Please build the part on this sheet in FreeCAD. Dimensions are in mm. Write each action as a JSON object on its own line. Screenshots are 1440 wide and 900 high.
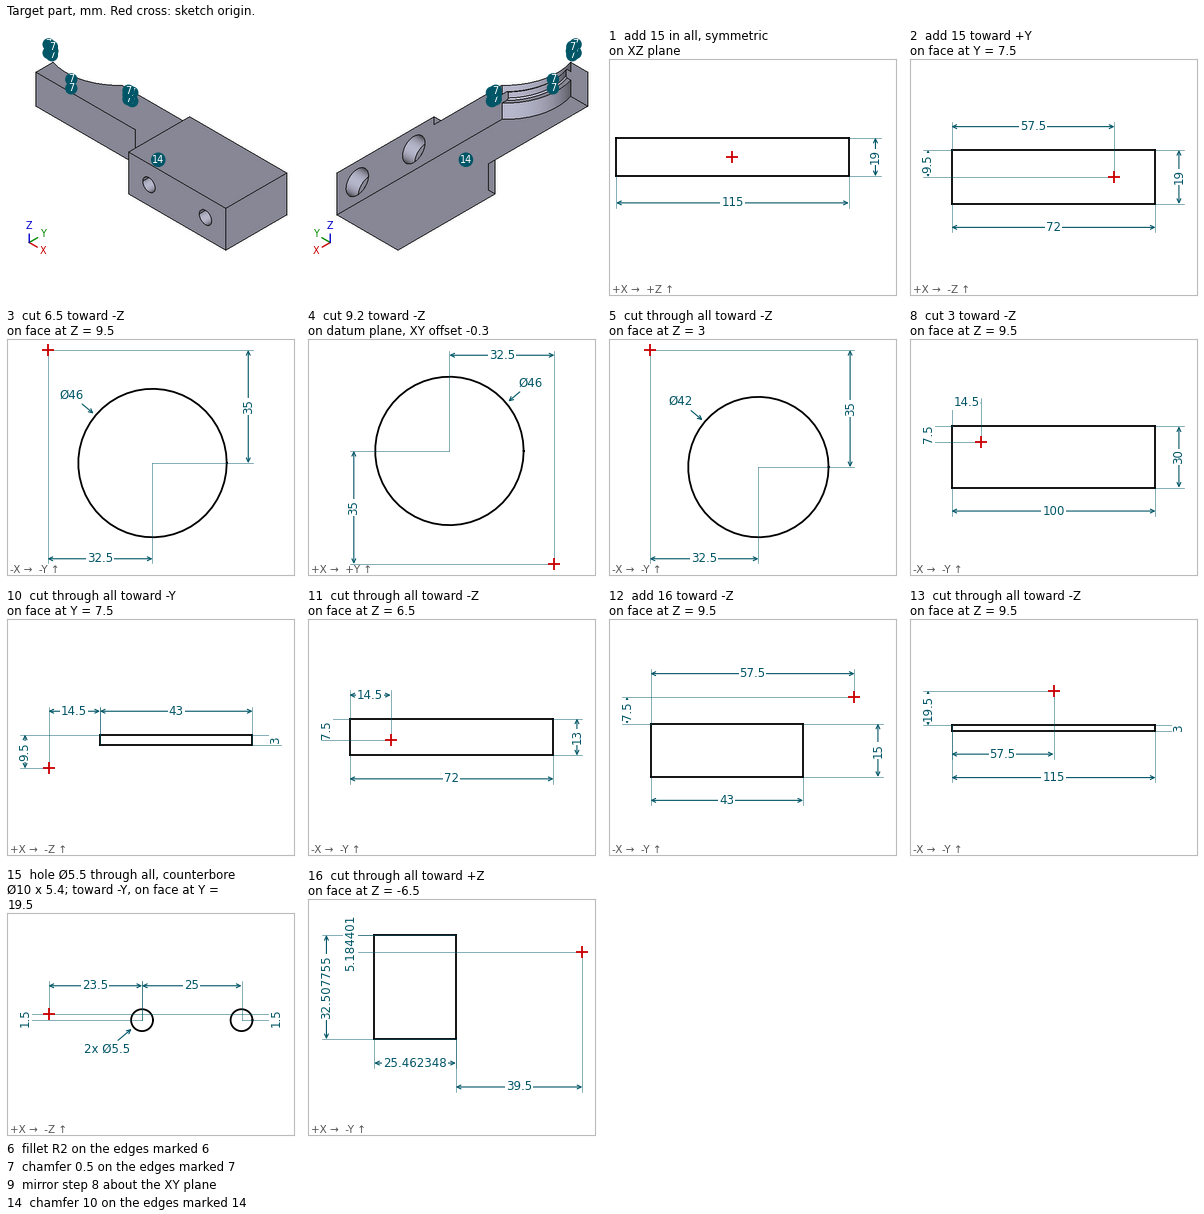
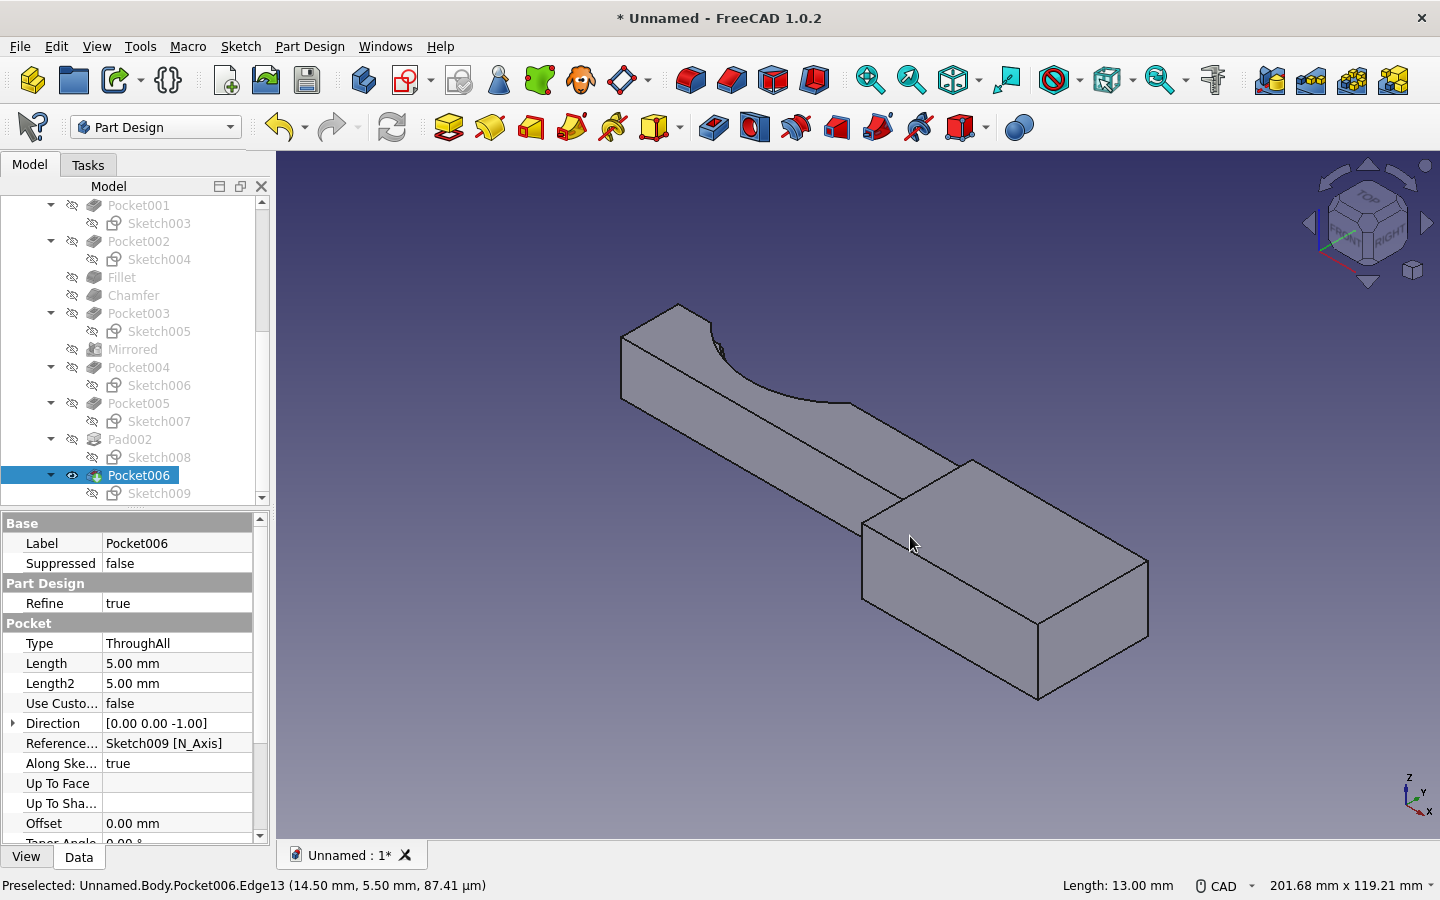
{"action": "left_click", "coordinate": [732, 80]}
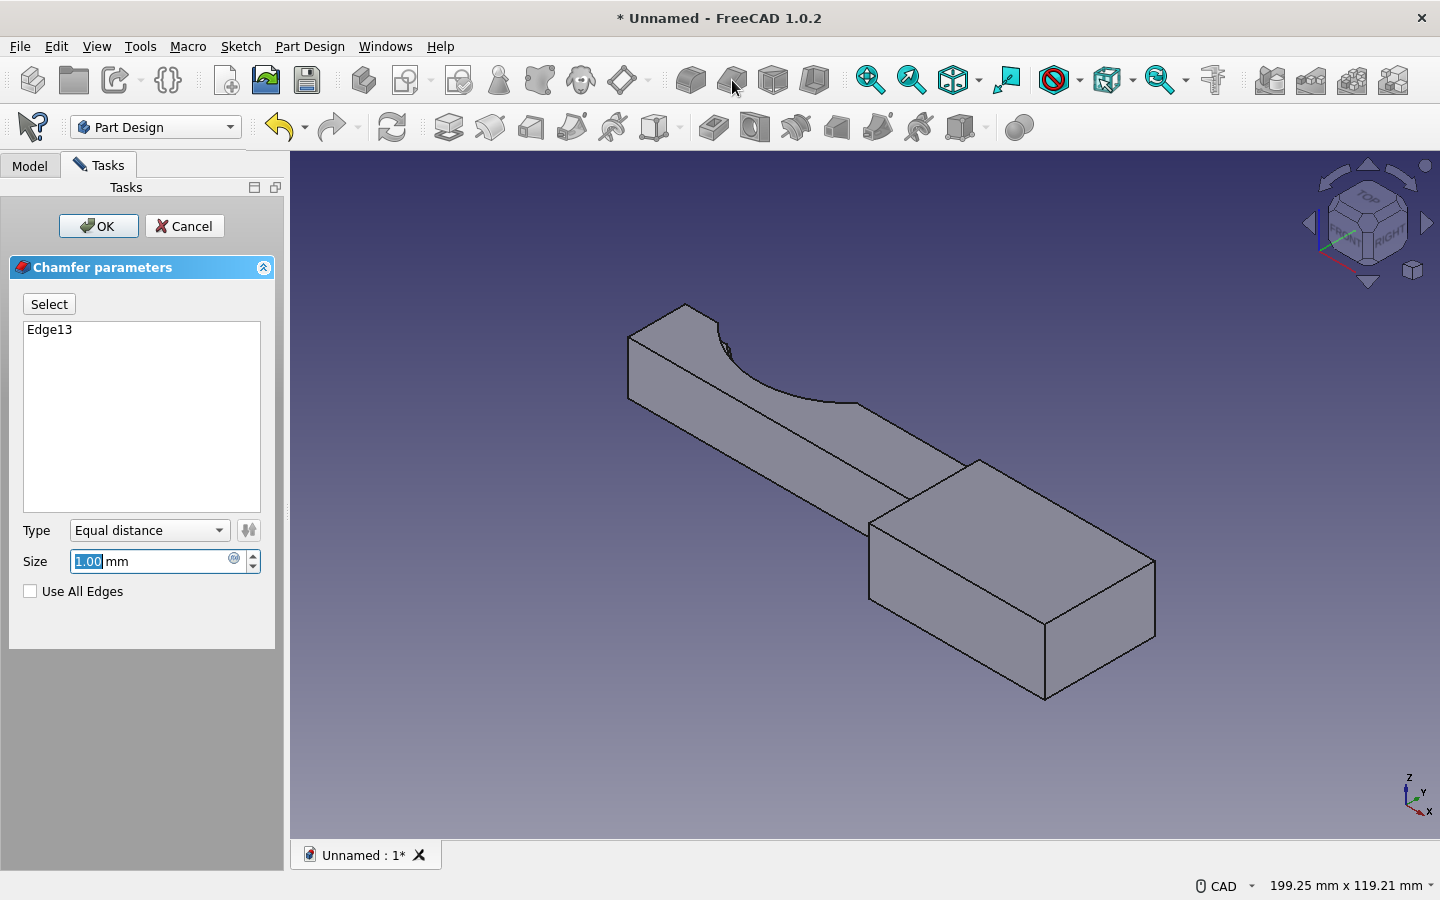
{"action": "type", "text": "10"}
{"action": "key", "text": "Tab"}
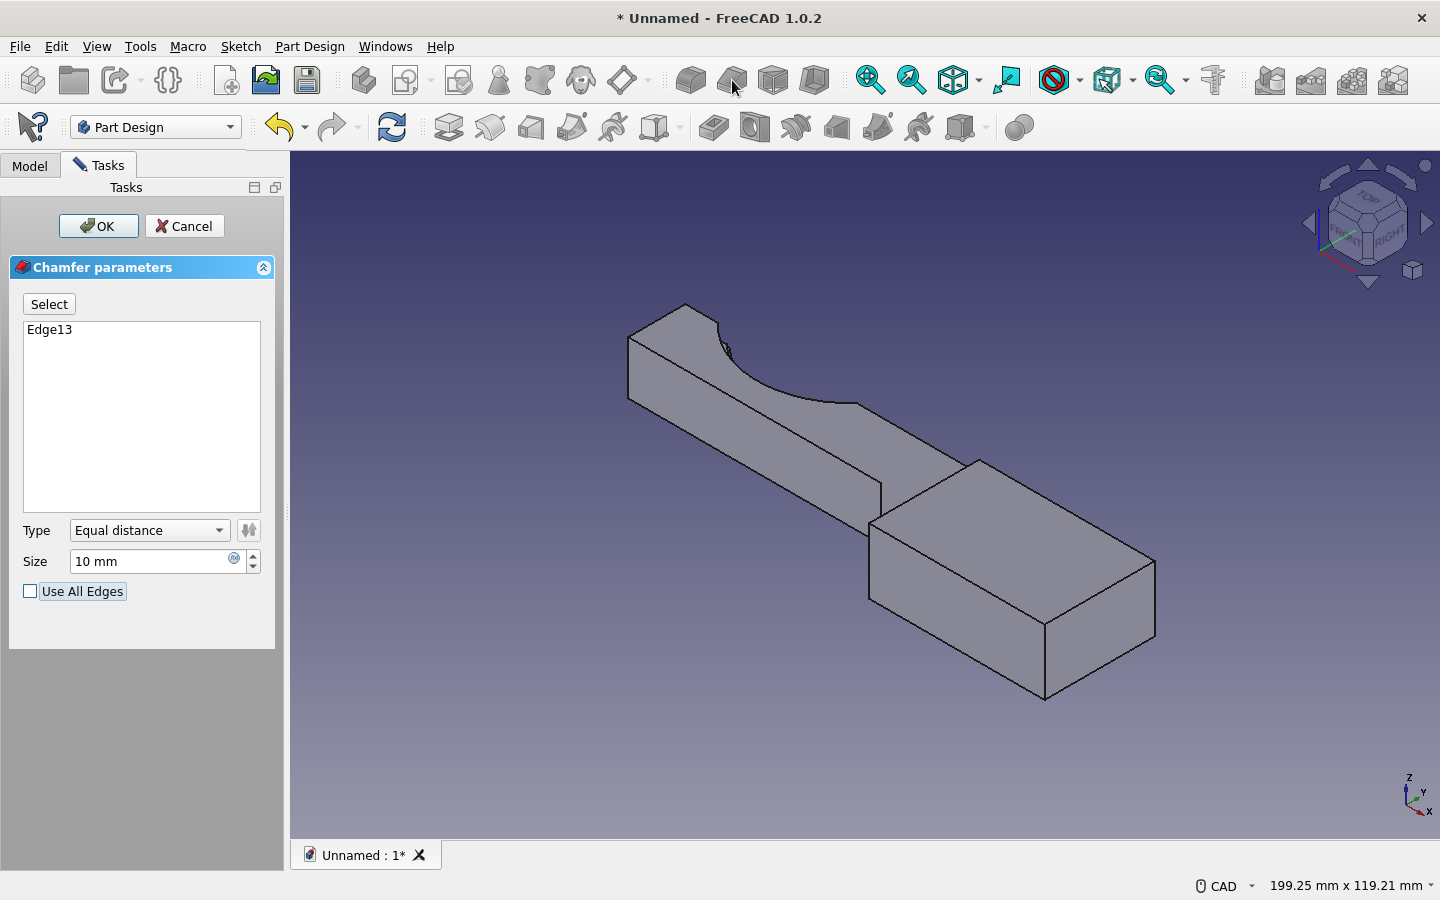
{"action": "left_click", "coordinate": [99, 226]}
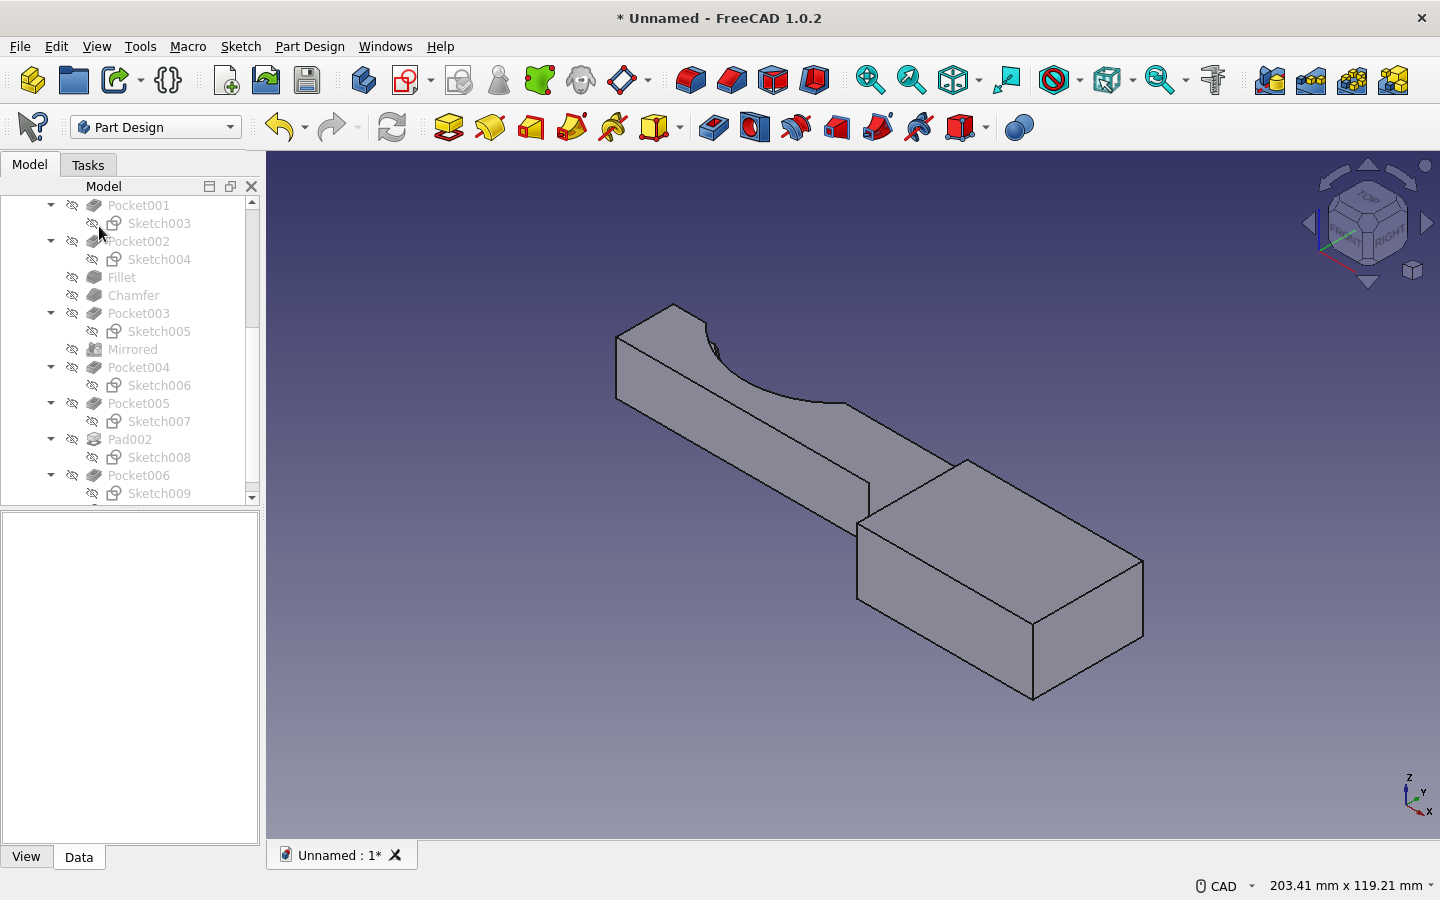
{"action": "key", "text": "4"}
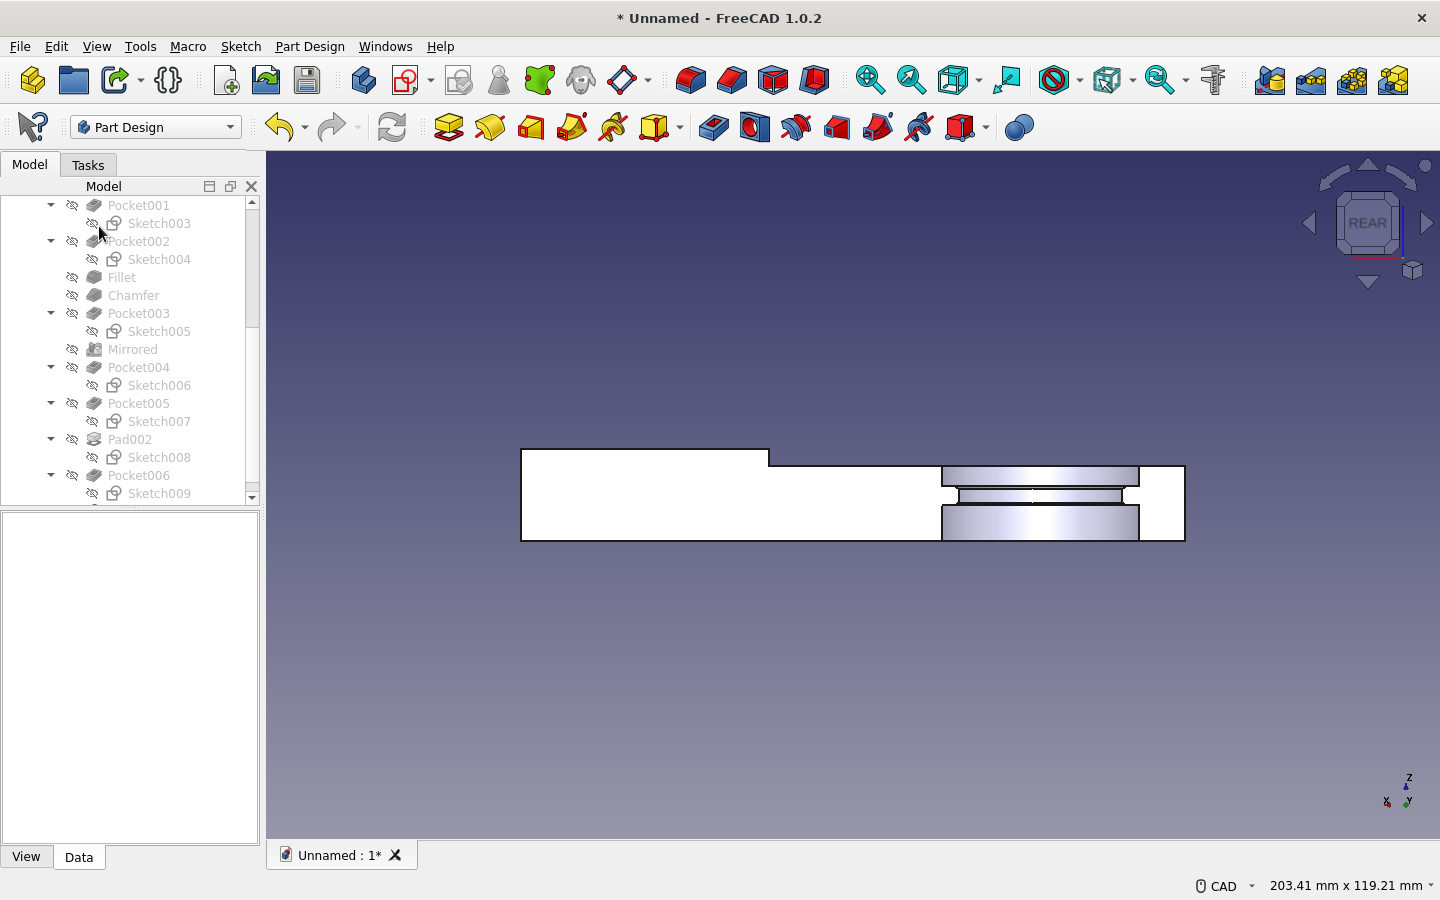
{"action": "left_click", "coordinate": [615, 494]}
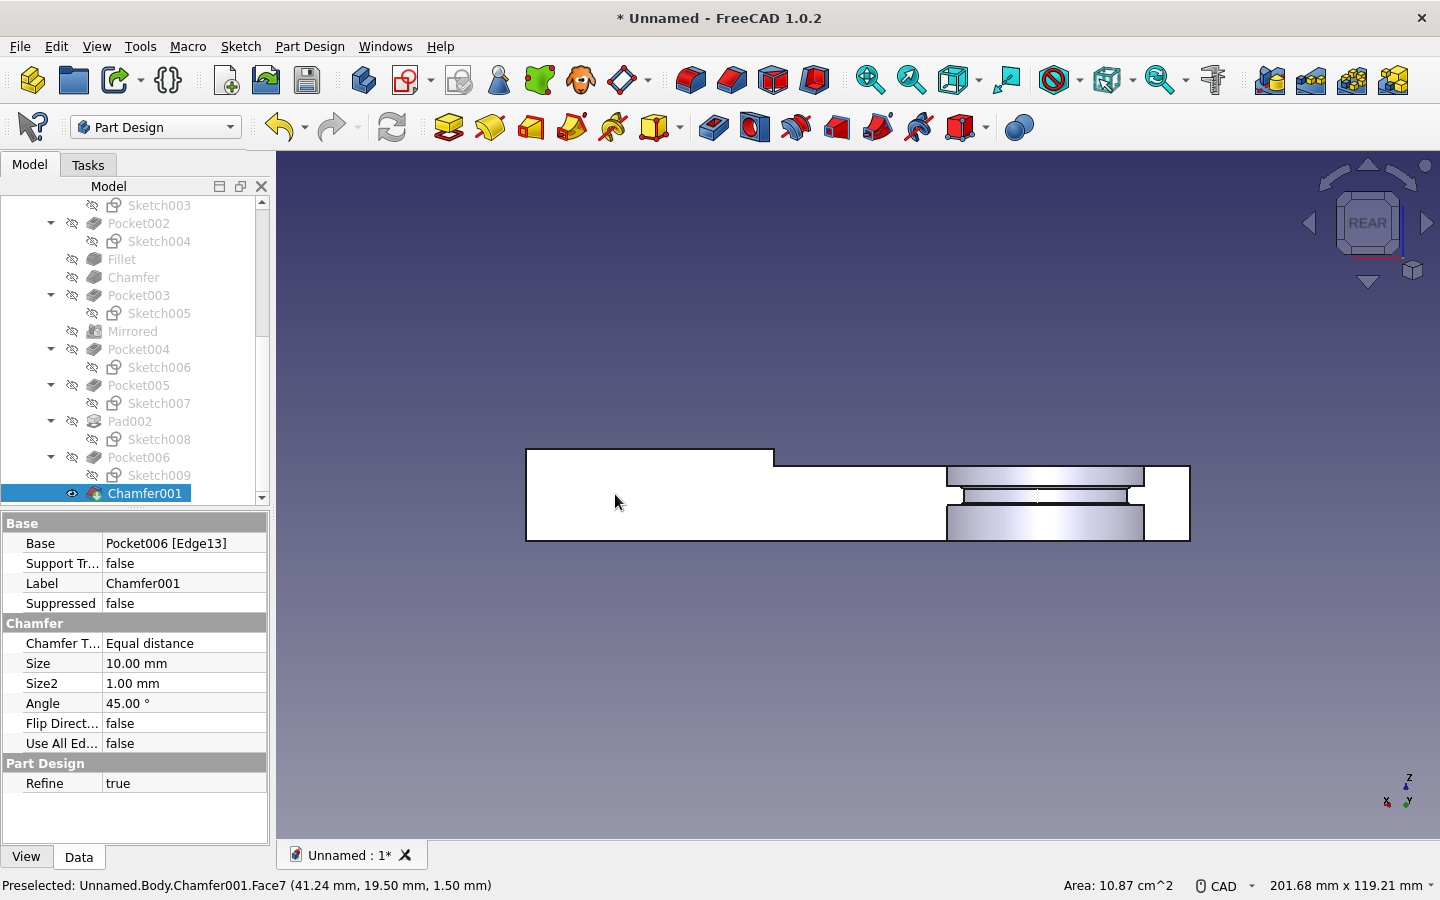
{"action": "left_click", "coordinate": [404, 80]}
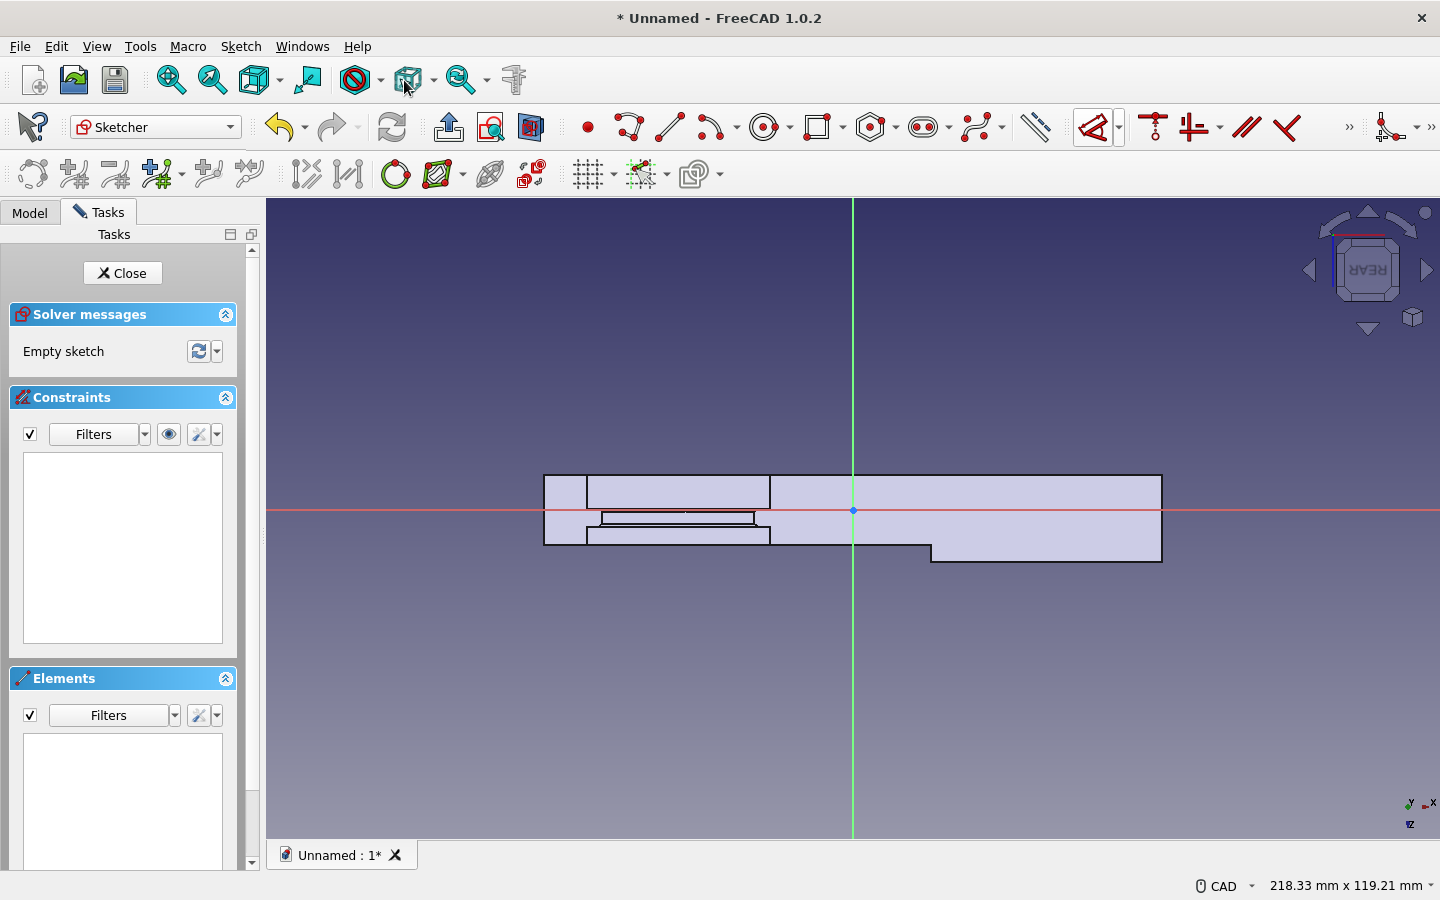
{"action": "scroll", "coordinate": [1111, 519], "scroll_direction": "up", "scroll_amount": 5}